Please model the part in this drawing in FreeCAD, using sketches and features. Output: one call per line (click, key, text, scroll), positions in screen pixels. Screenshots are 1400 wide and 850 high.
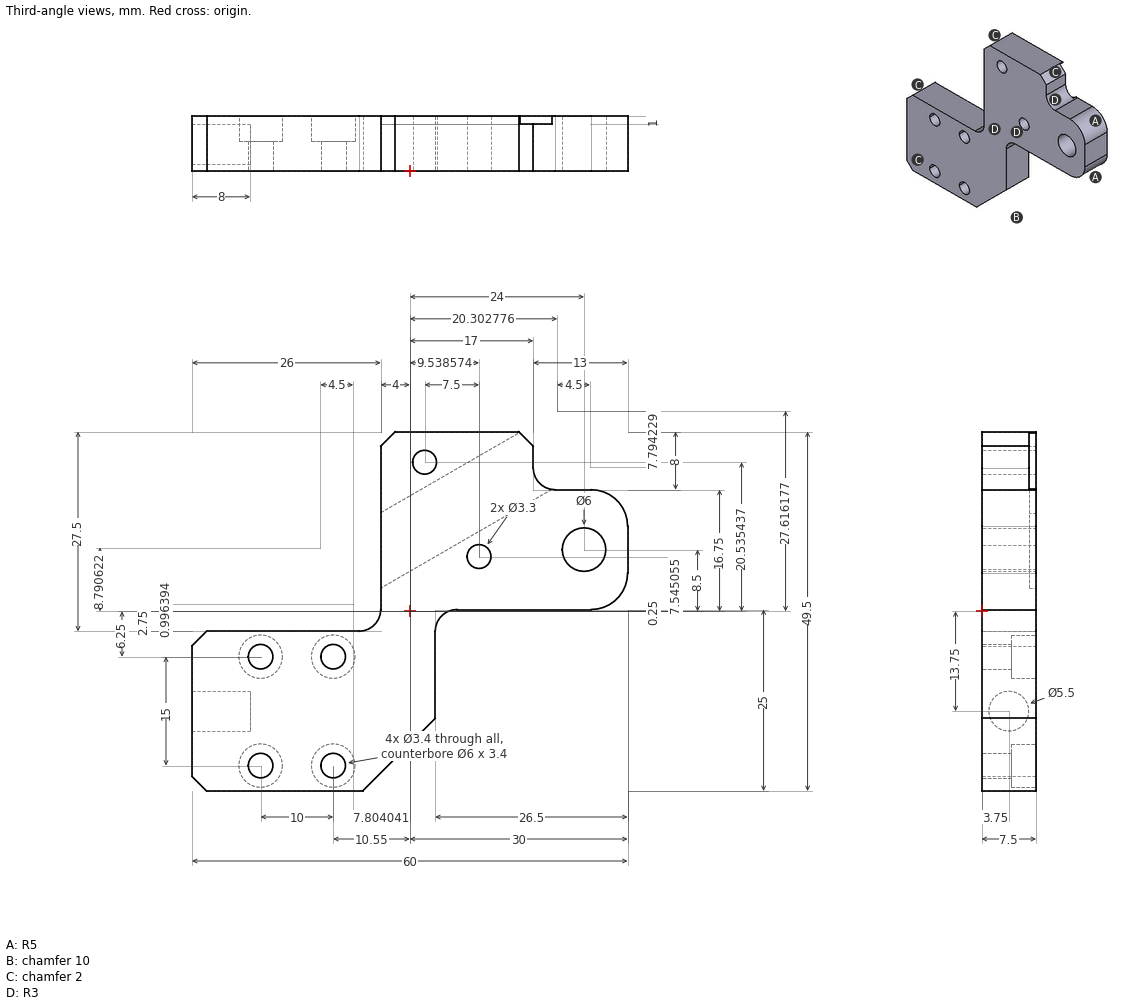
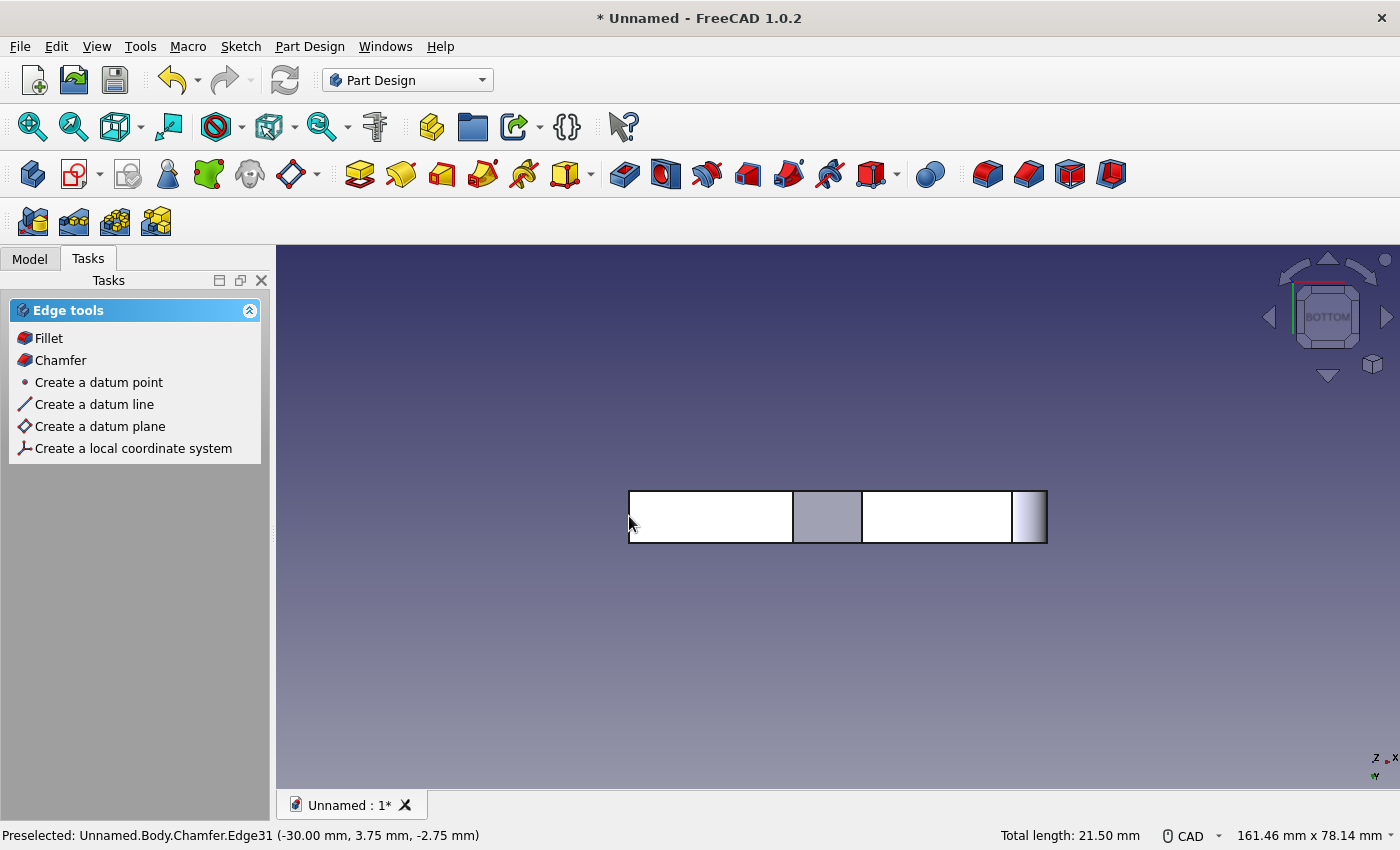
click(629, 516, ctrl)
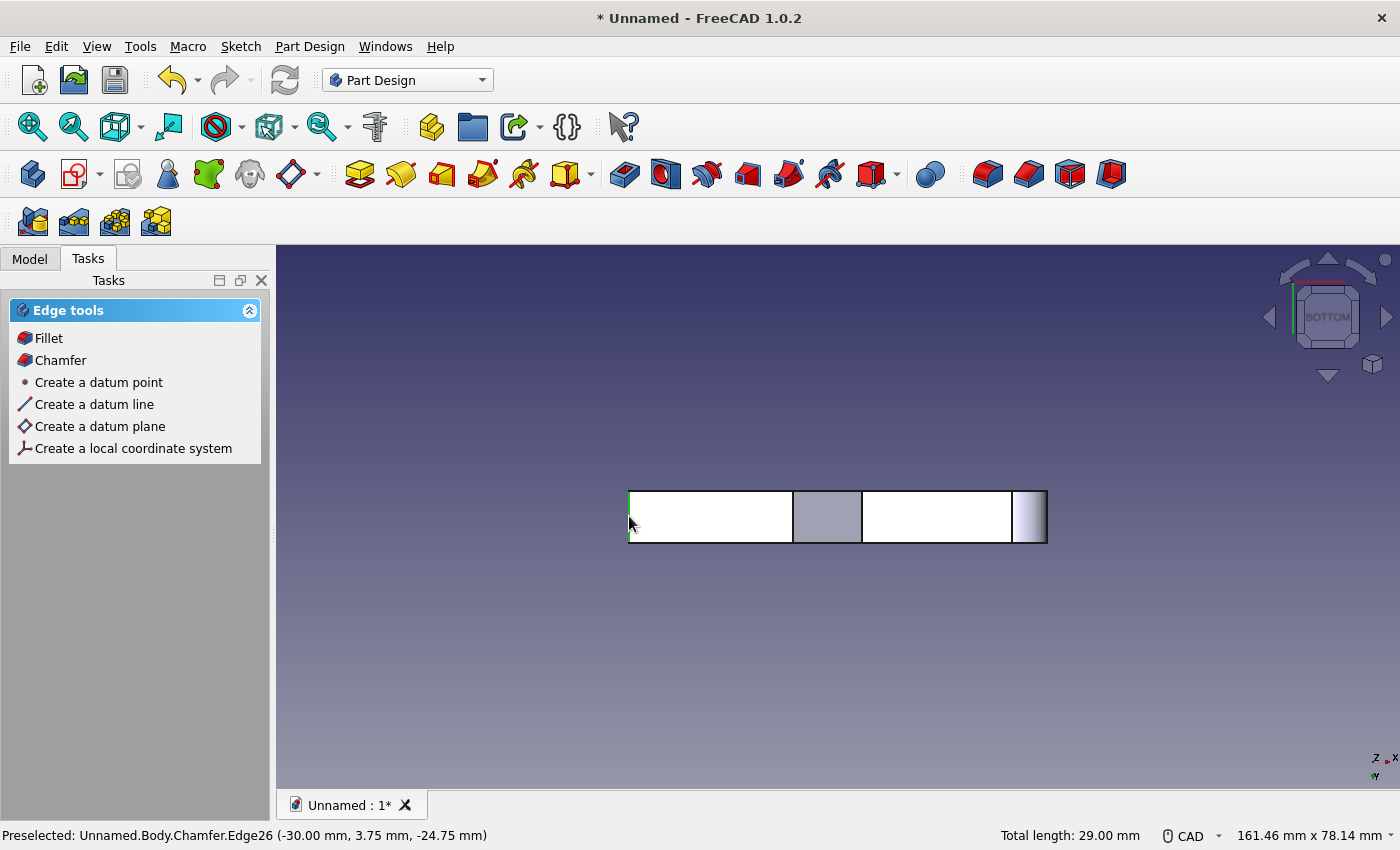
click(1029, 174)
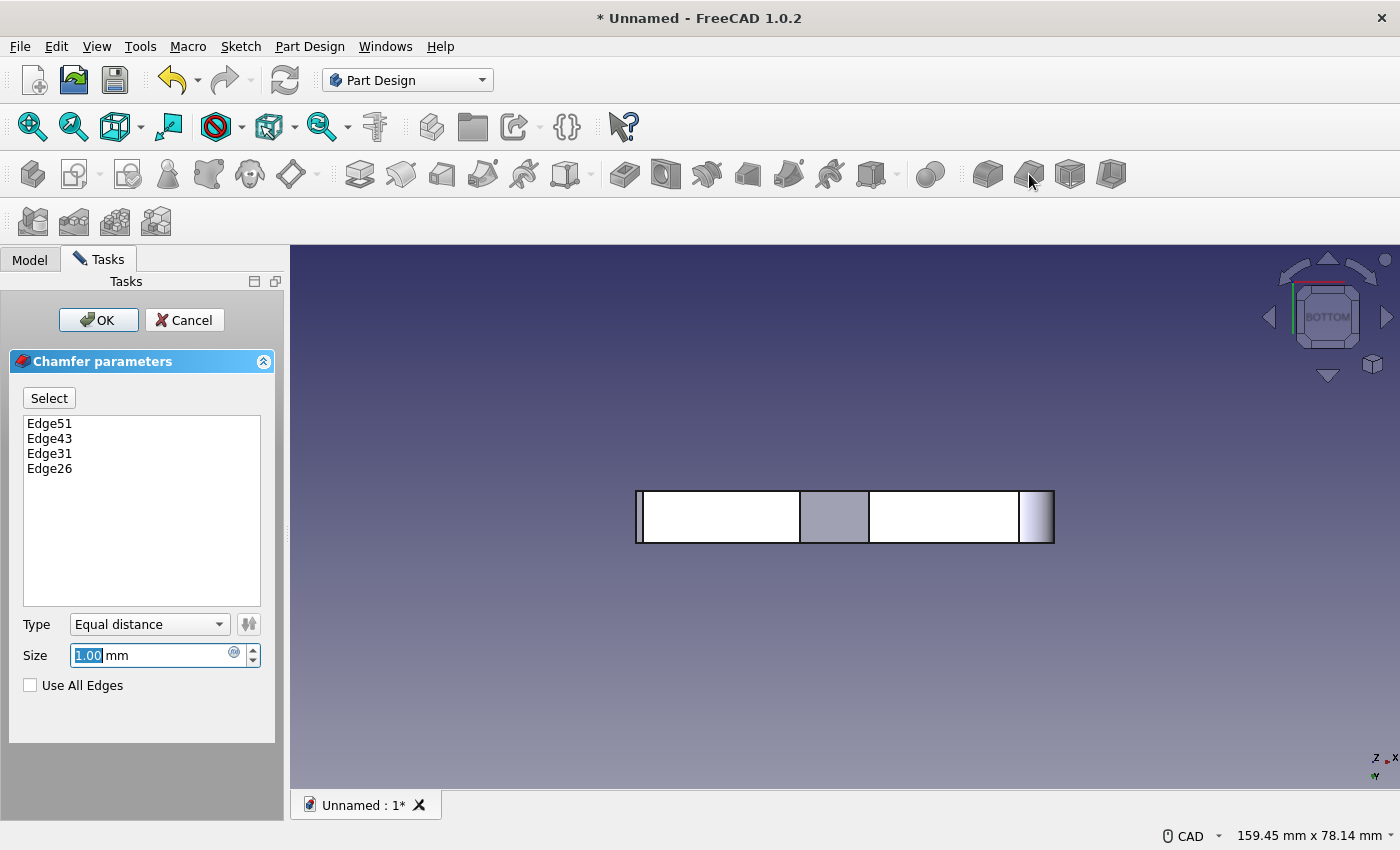
text(2)
key(Tab)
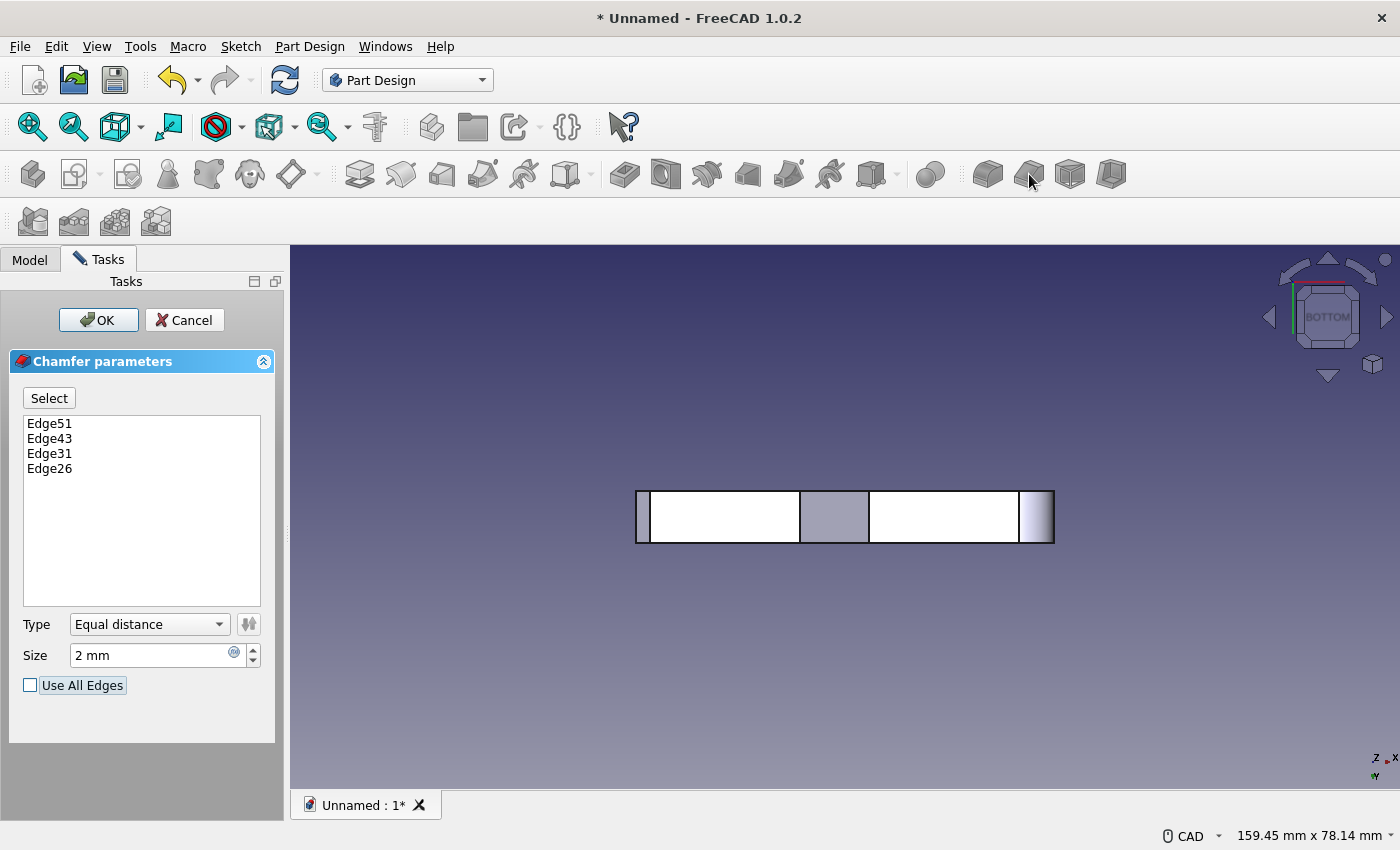
click(99, 320)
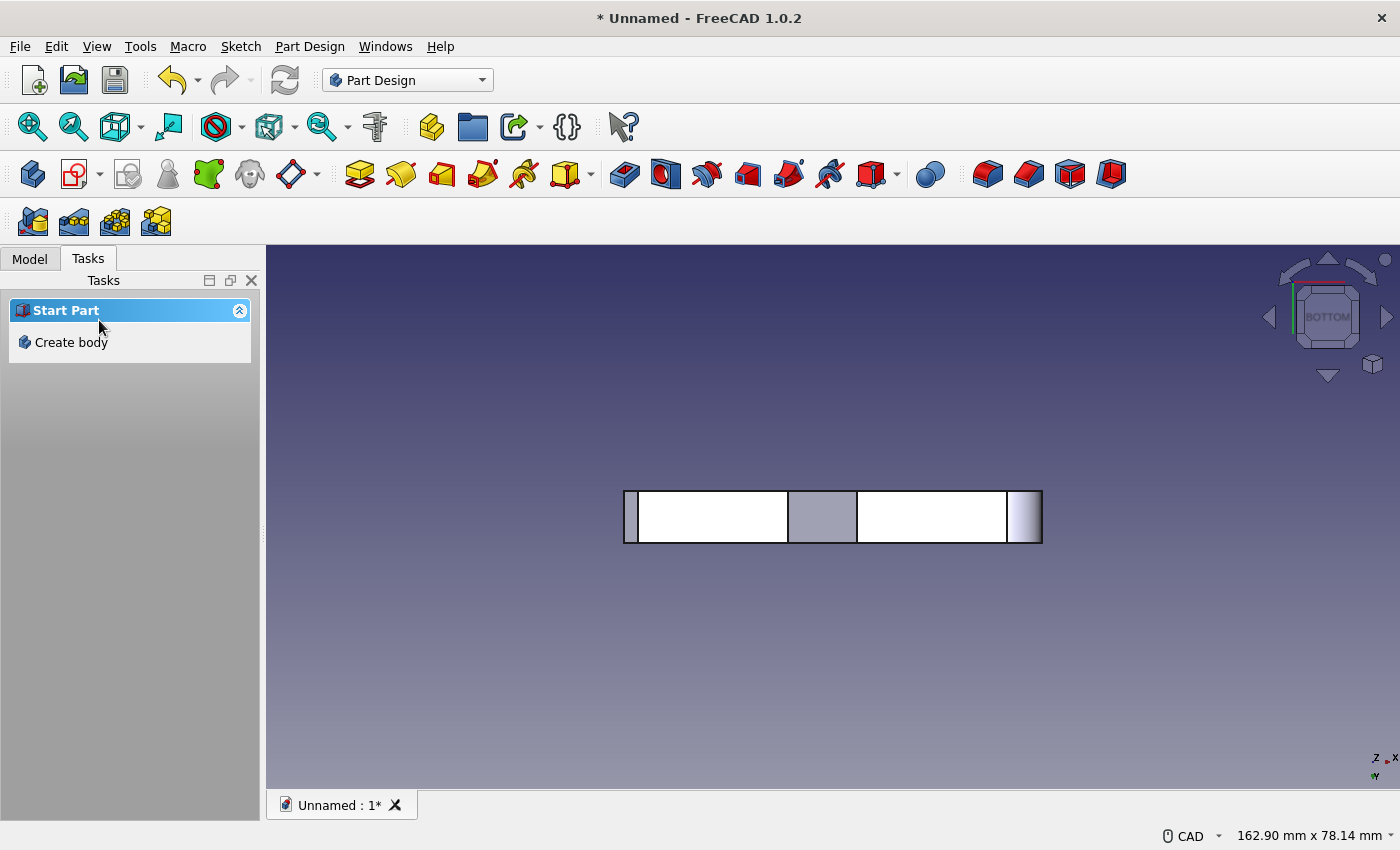
key(v)
key(f)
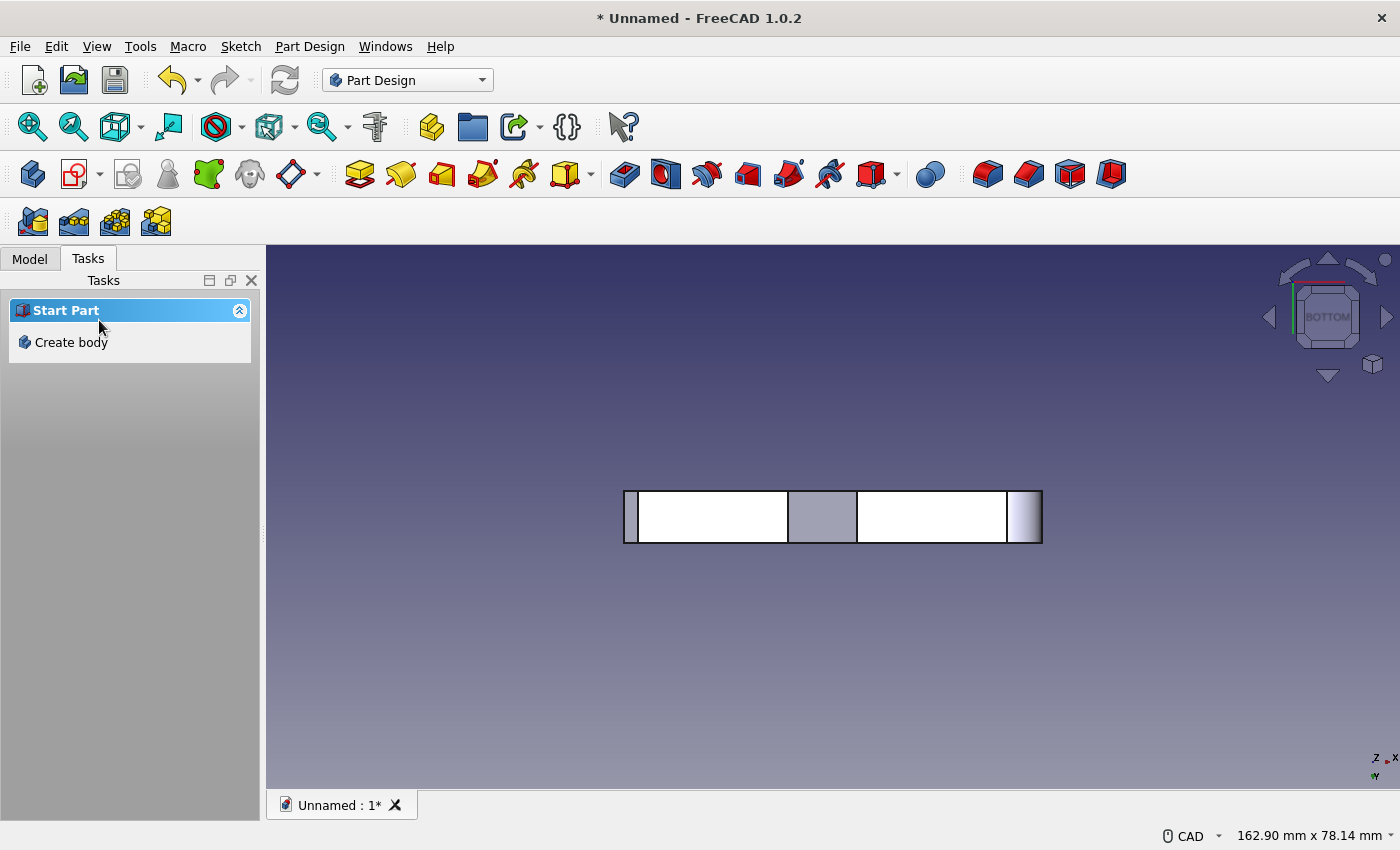
key(0)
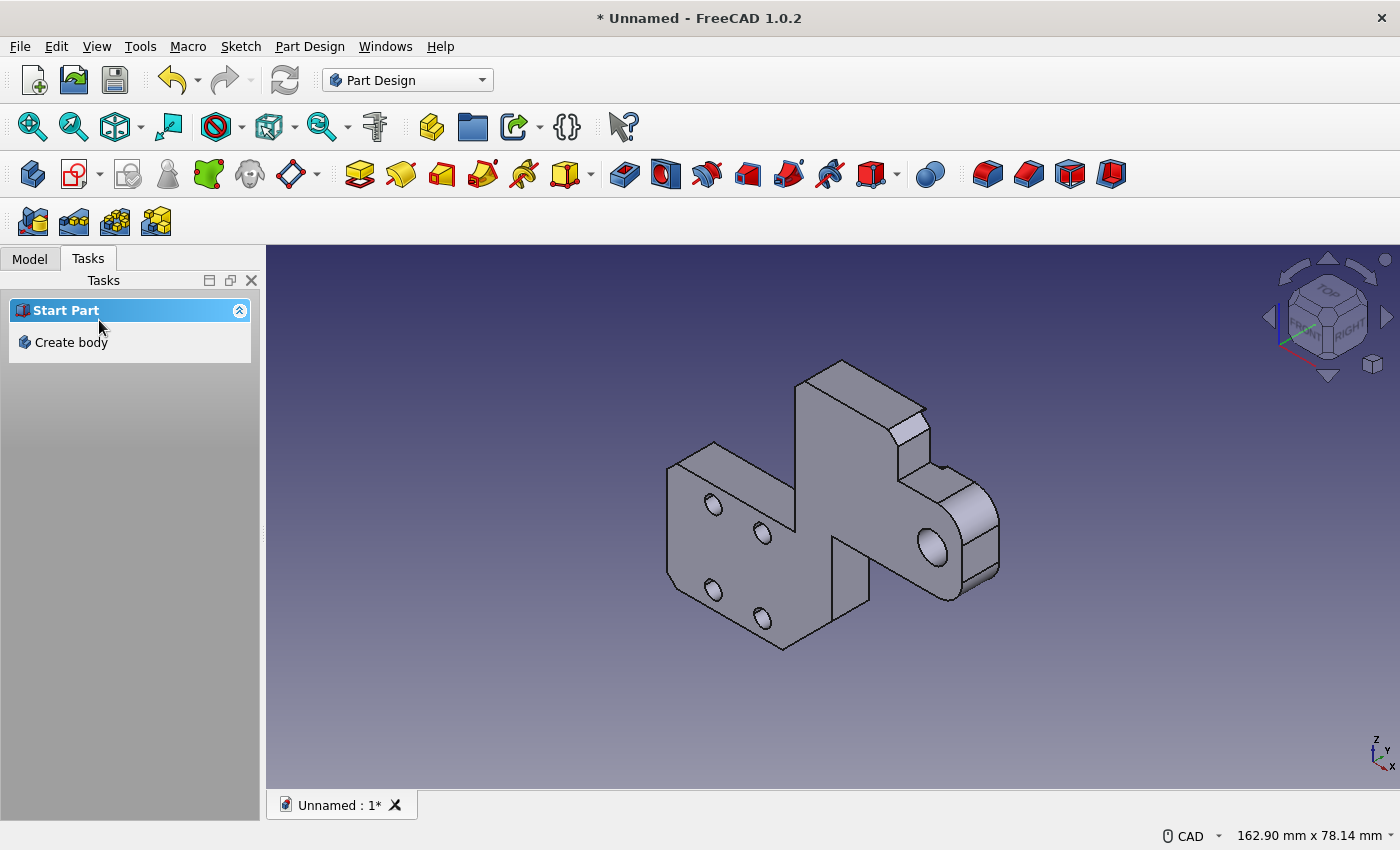
key(2)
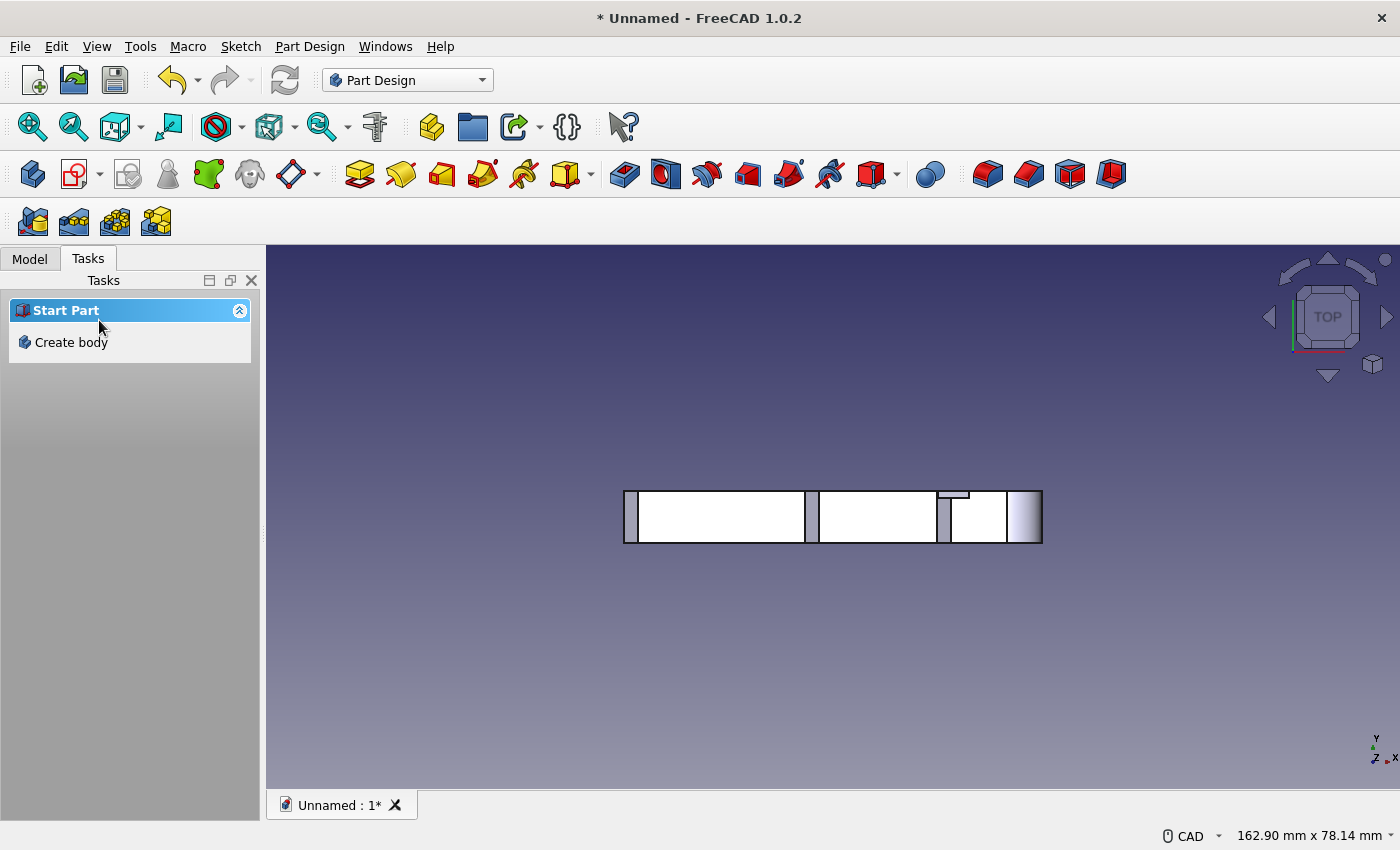
key(v)
key(f)